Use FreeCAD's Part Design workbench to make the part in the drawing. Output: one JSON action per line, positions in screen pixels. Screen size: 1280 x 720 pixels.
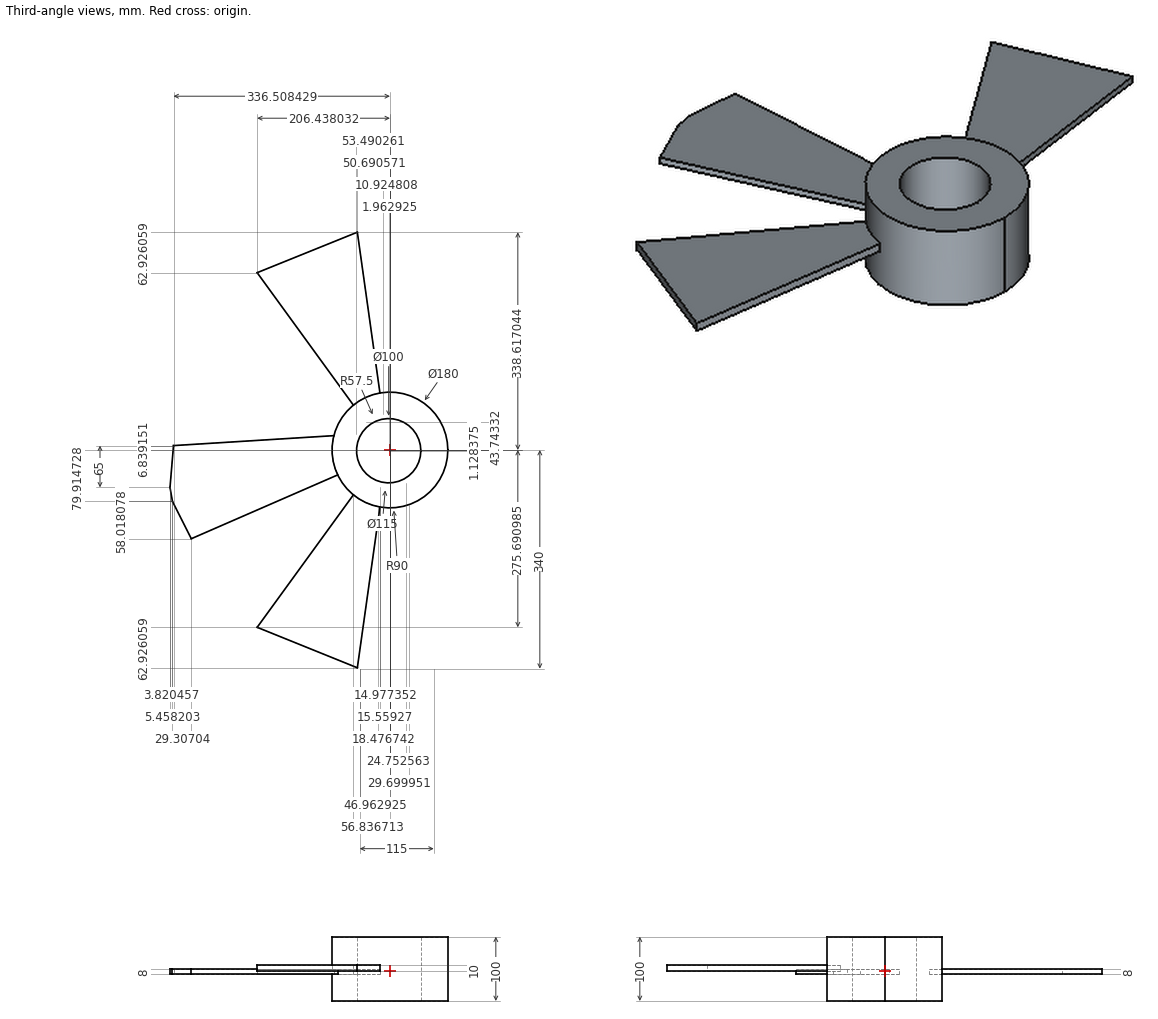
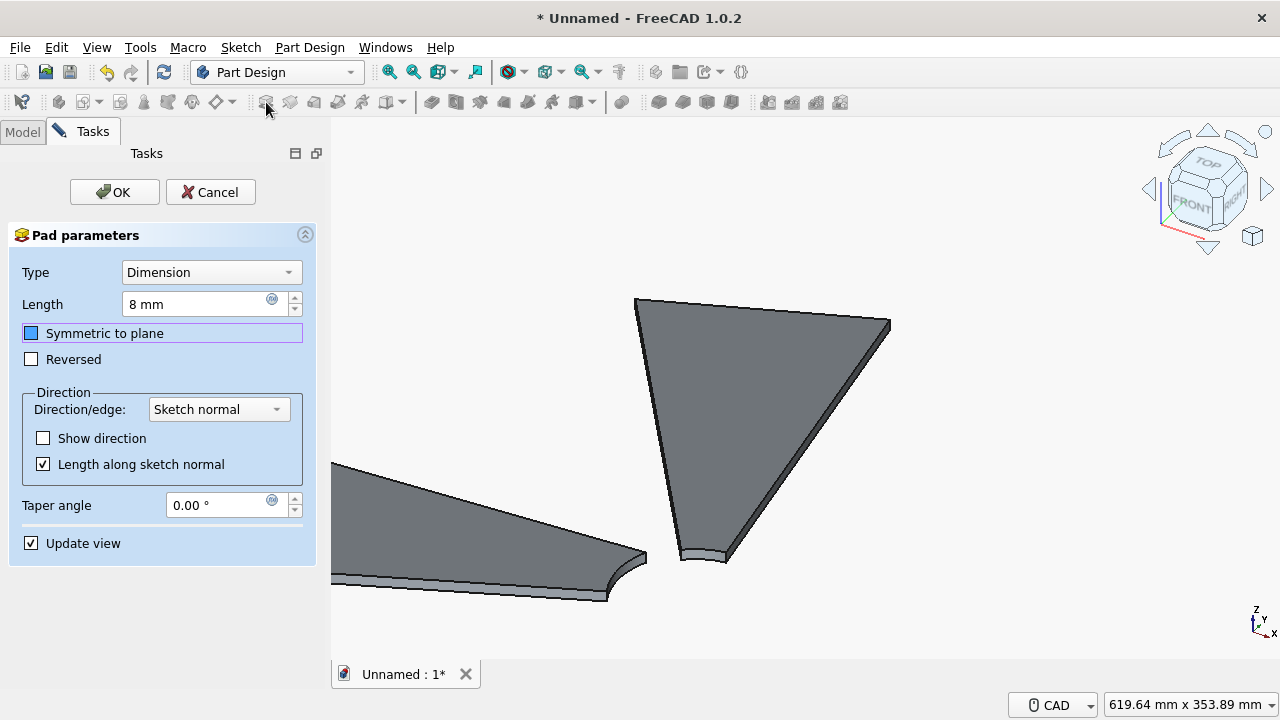
{"action": "left_click", "coordinate": [30, 333]}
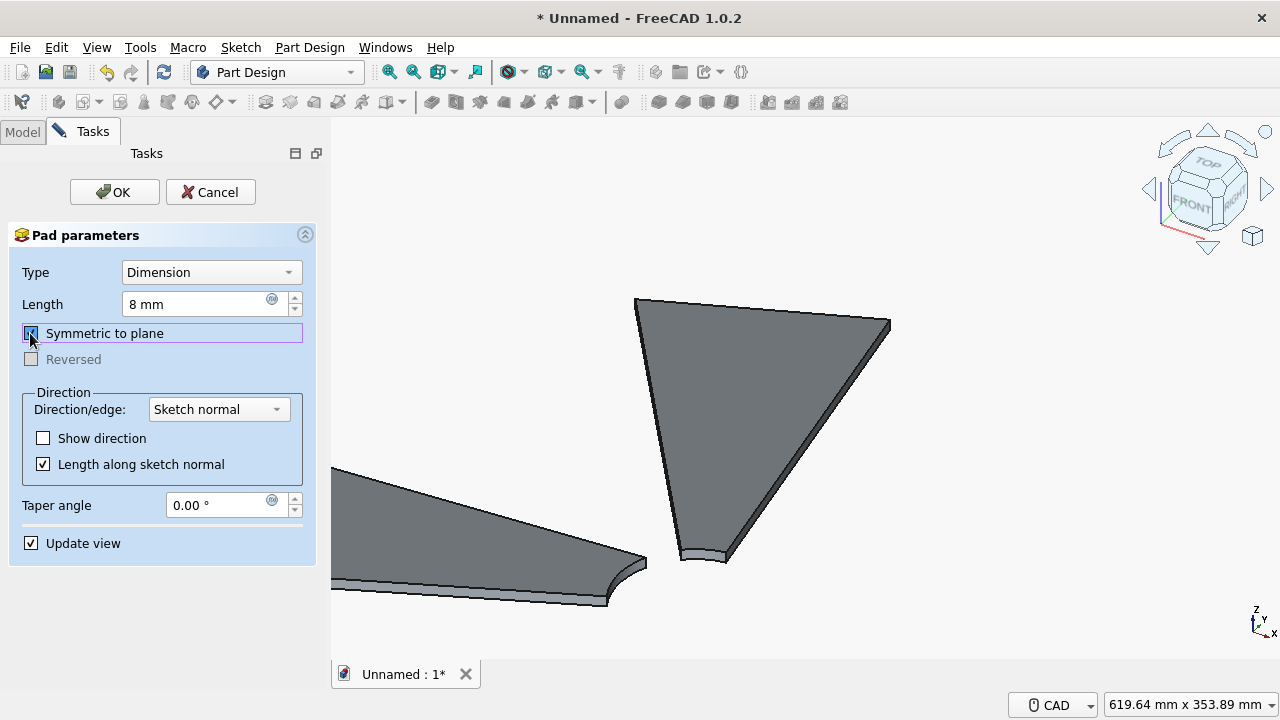
{"action": "left_click", "coordinate": [115, 192]}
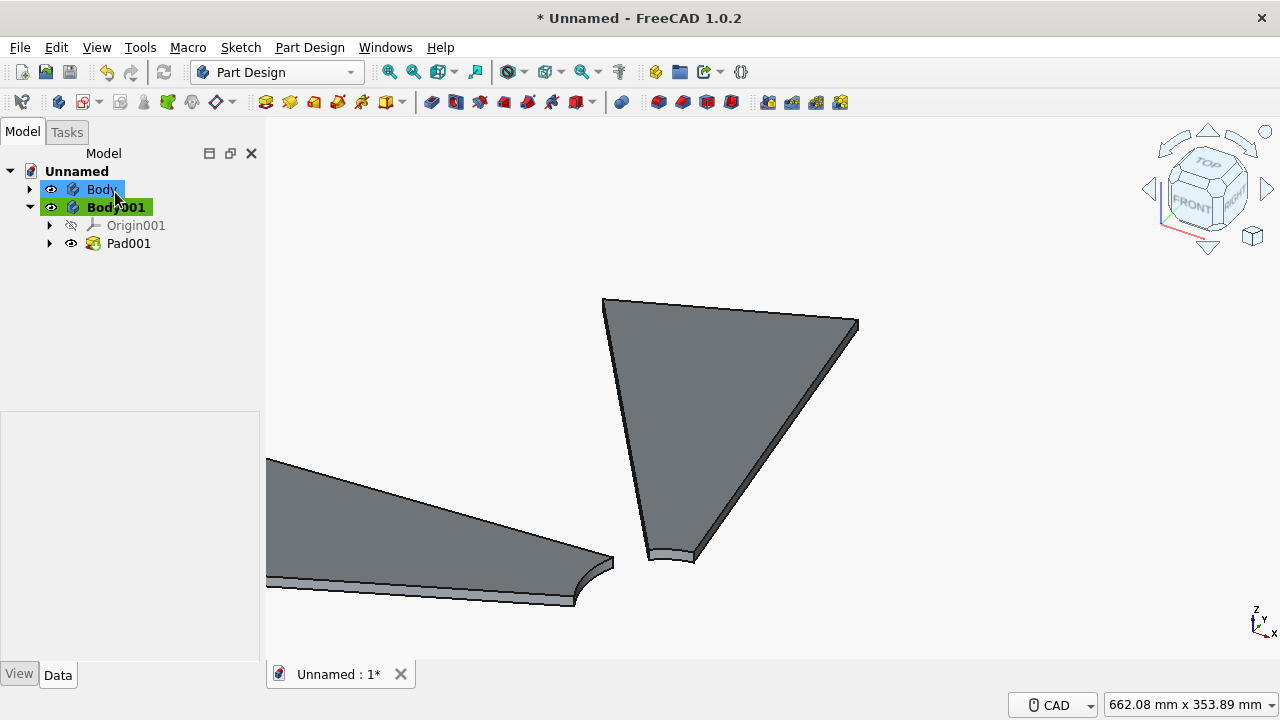
{"action": "left_click", "coordinate": [390, 72]}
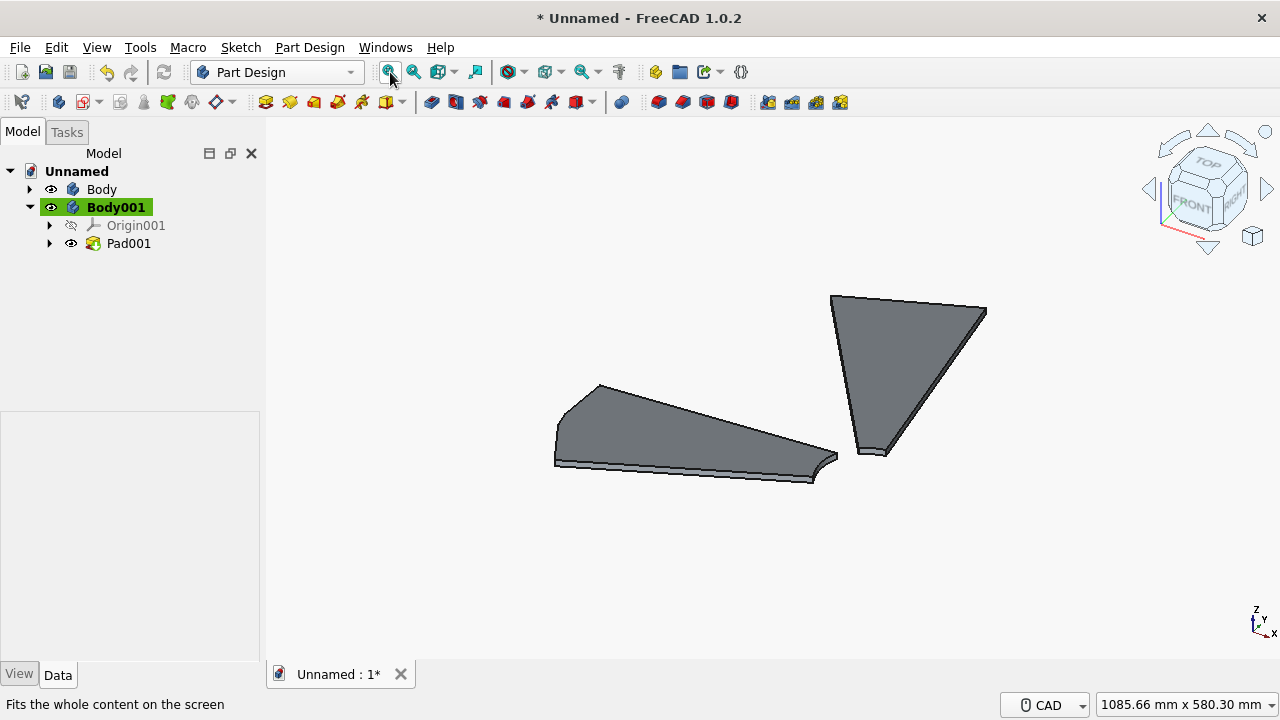
{"action": "left_click", "coordinate": [60, 102]}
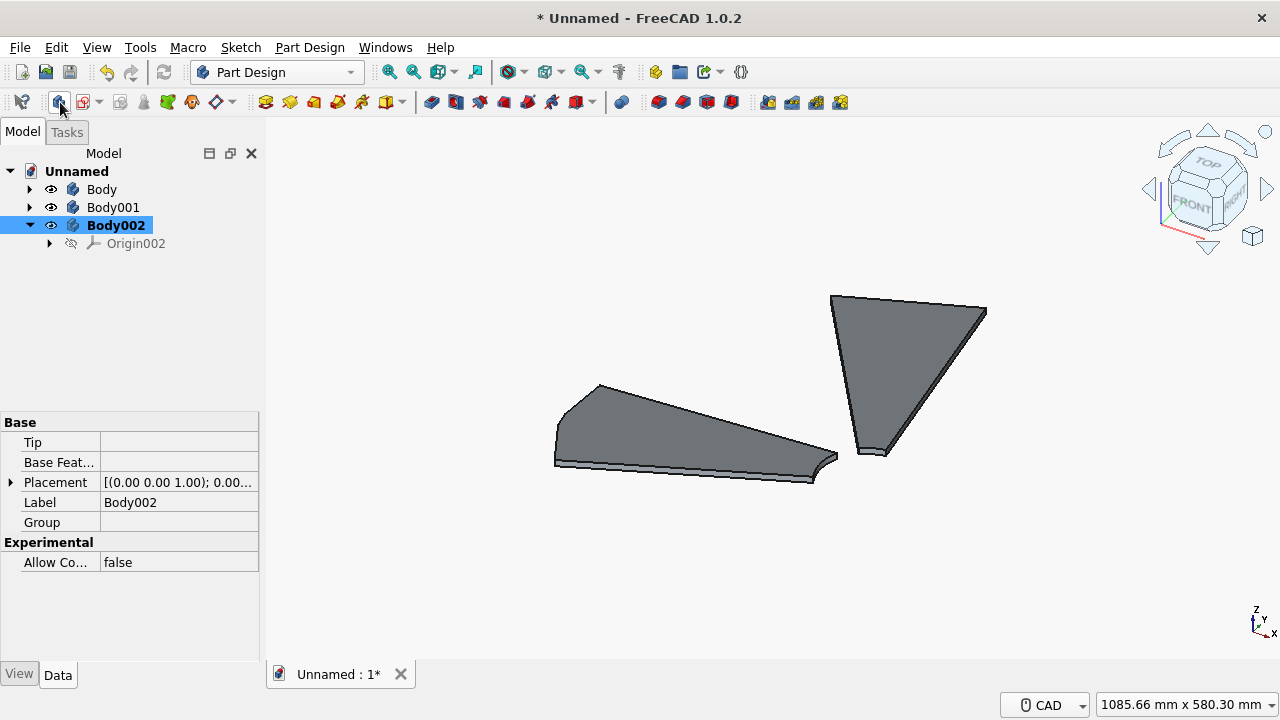
{"action": "left_click", "coordinate": [306, 619]}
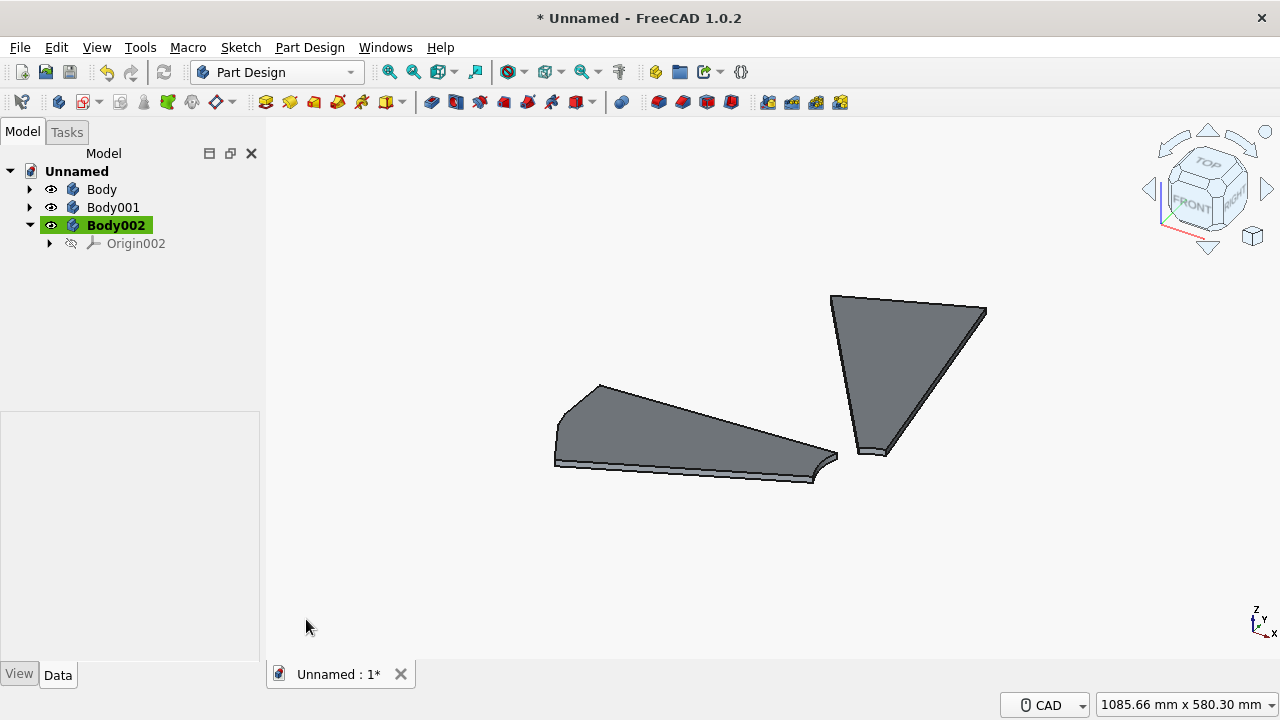
{"action": "left_click", "coordinate": [84, 102]}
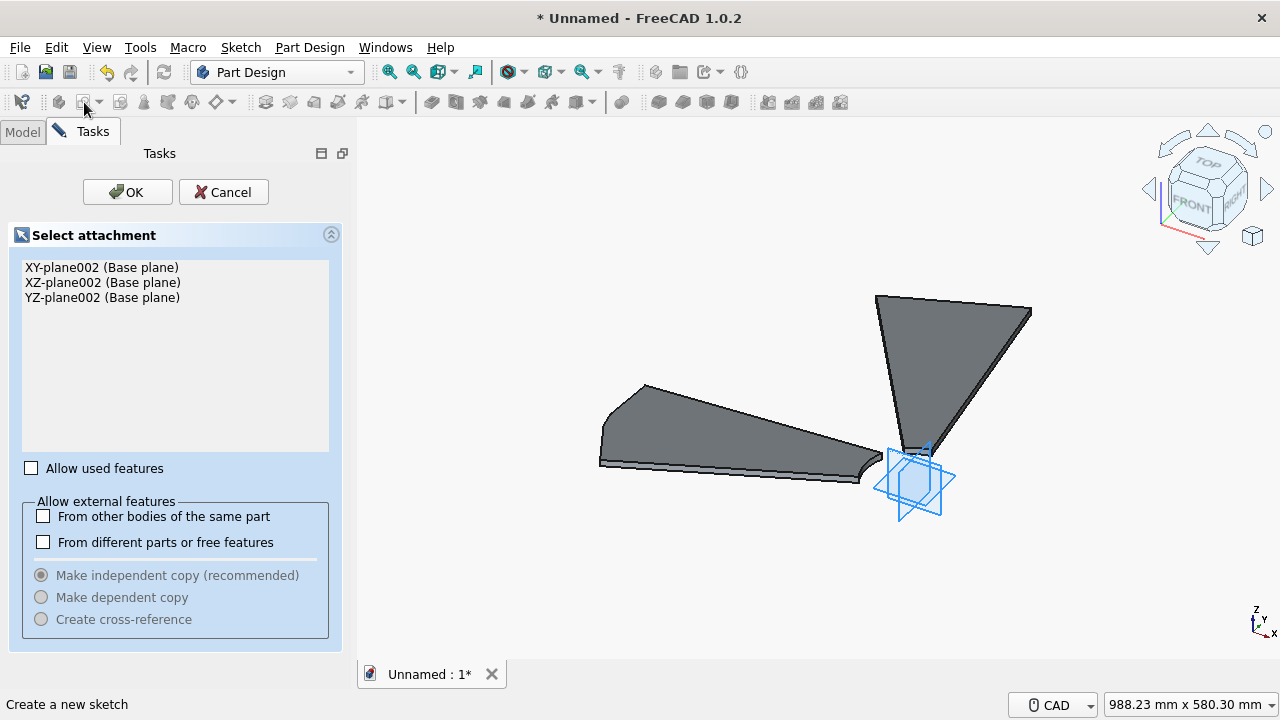
{"action": "left_click", "coordinate": [82, 268]}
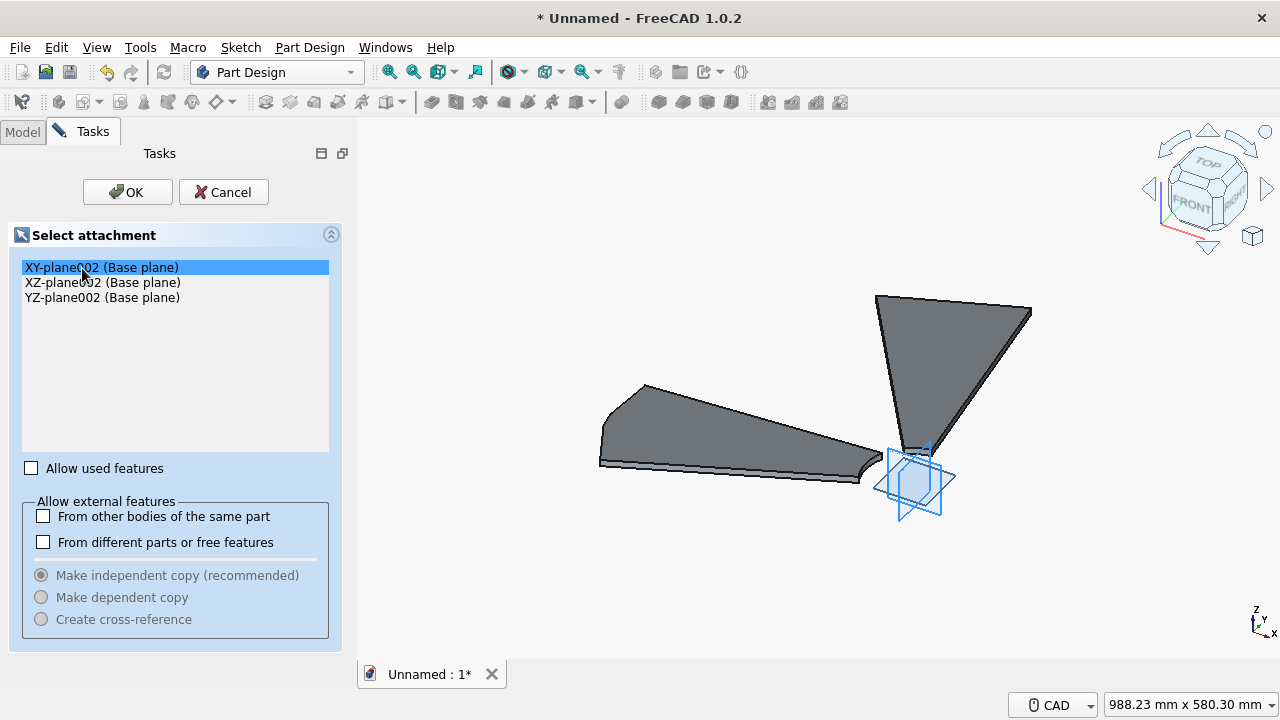
{"action": "left_click", "coordinate": [128, 192]}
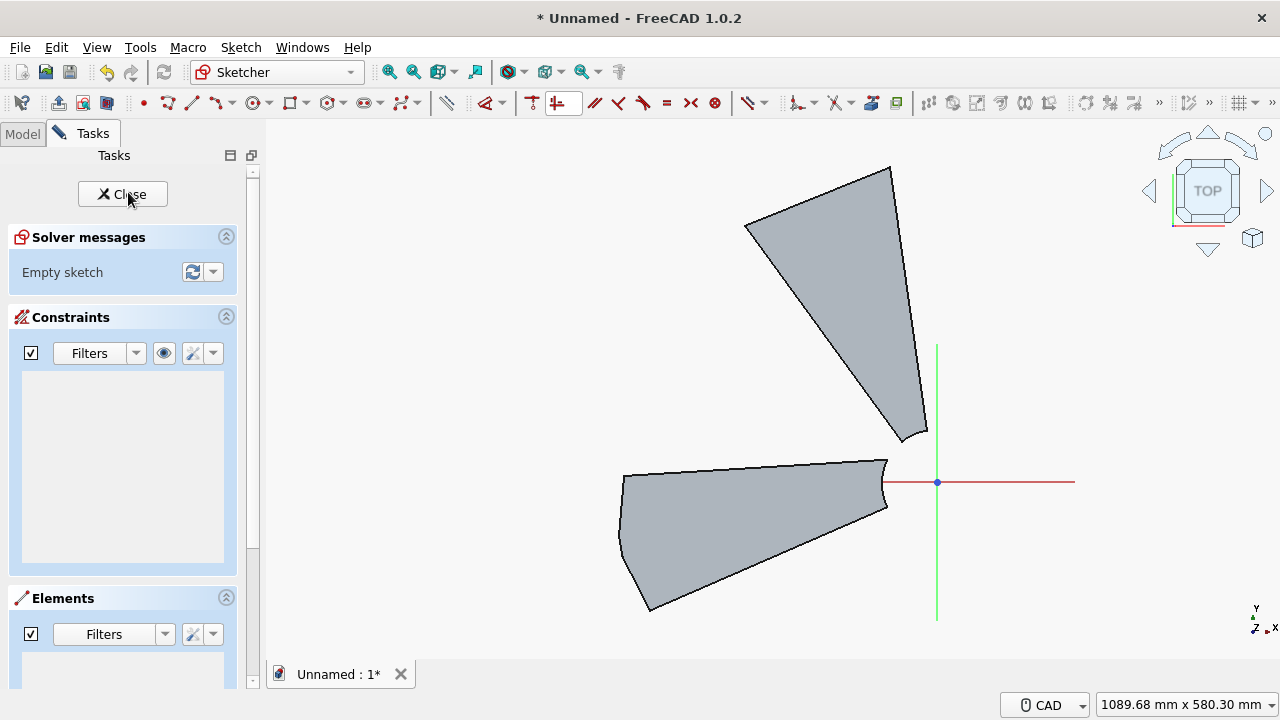
{"action": "scroll", "coordinate": [294, 147], "scroll_direction": "down", "scroll_amount": 2}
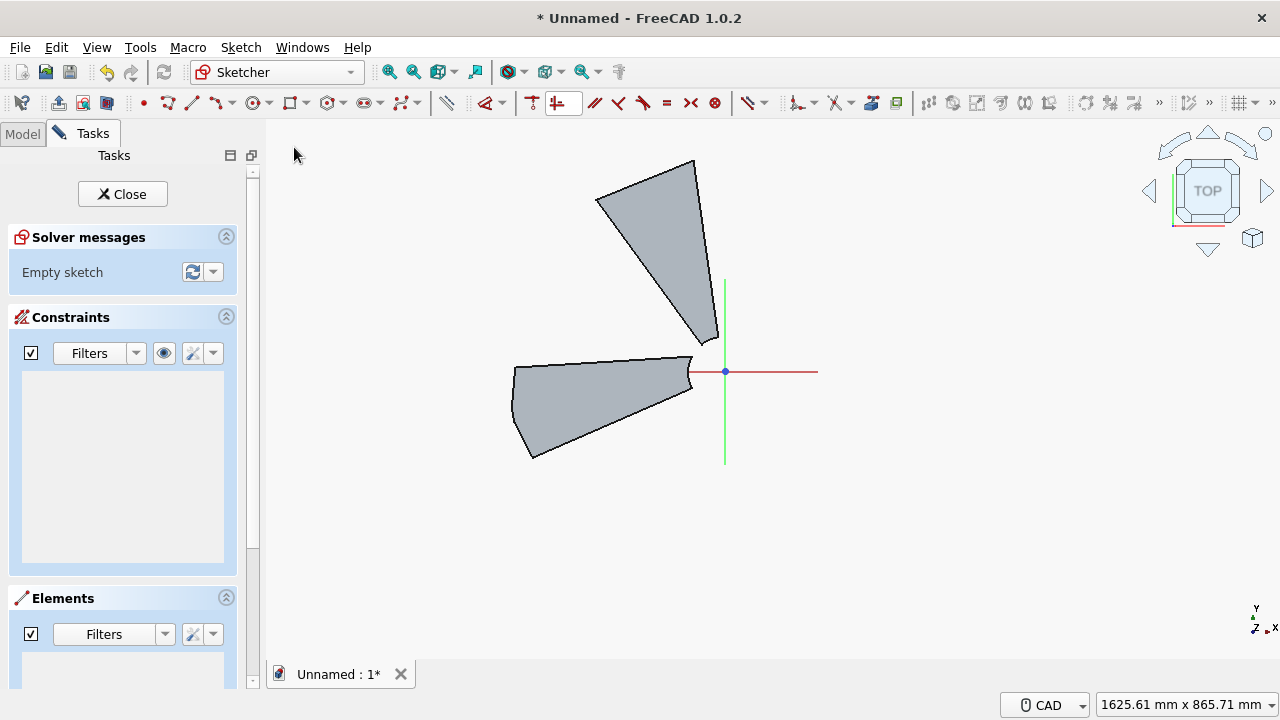
{"action": "scroll", "coordinate": [787, 631], "scroll_direction": "up", "scroll_amount": 2}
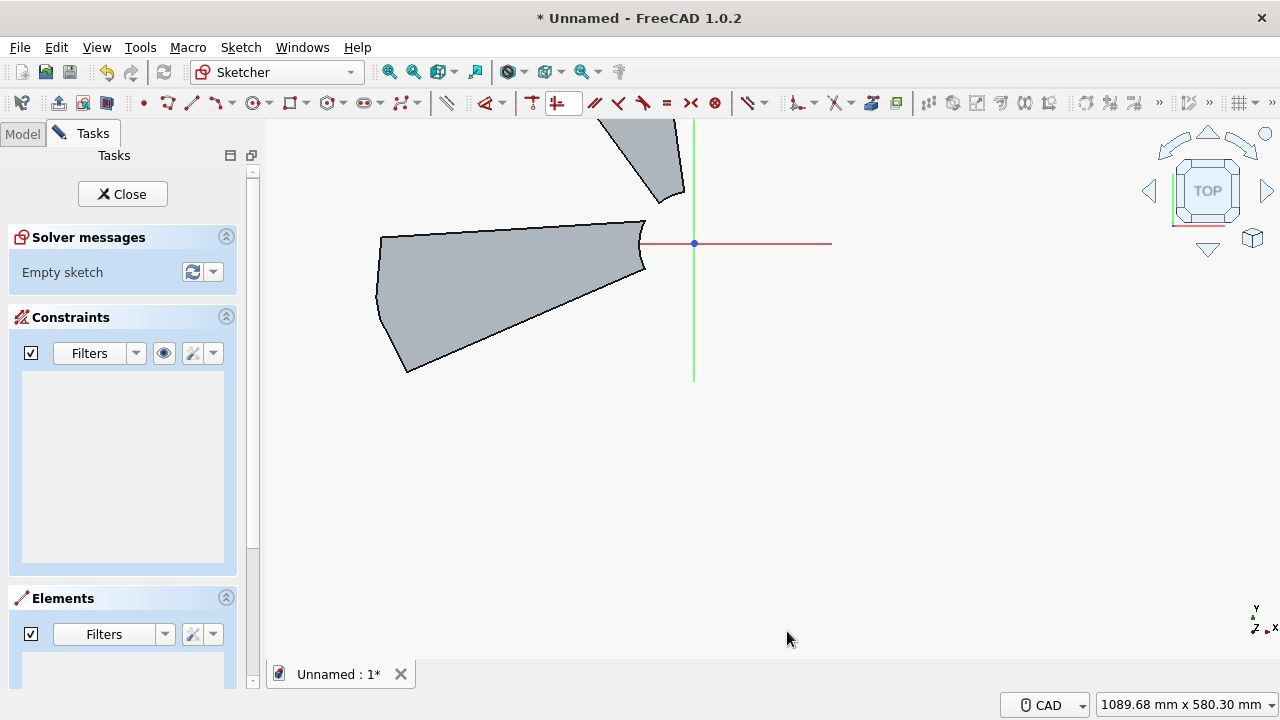
{"action": "left_click", "coordinate": [168, 104]}